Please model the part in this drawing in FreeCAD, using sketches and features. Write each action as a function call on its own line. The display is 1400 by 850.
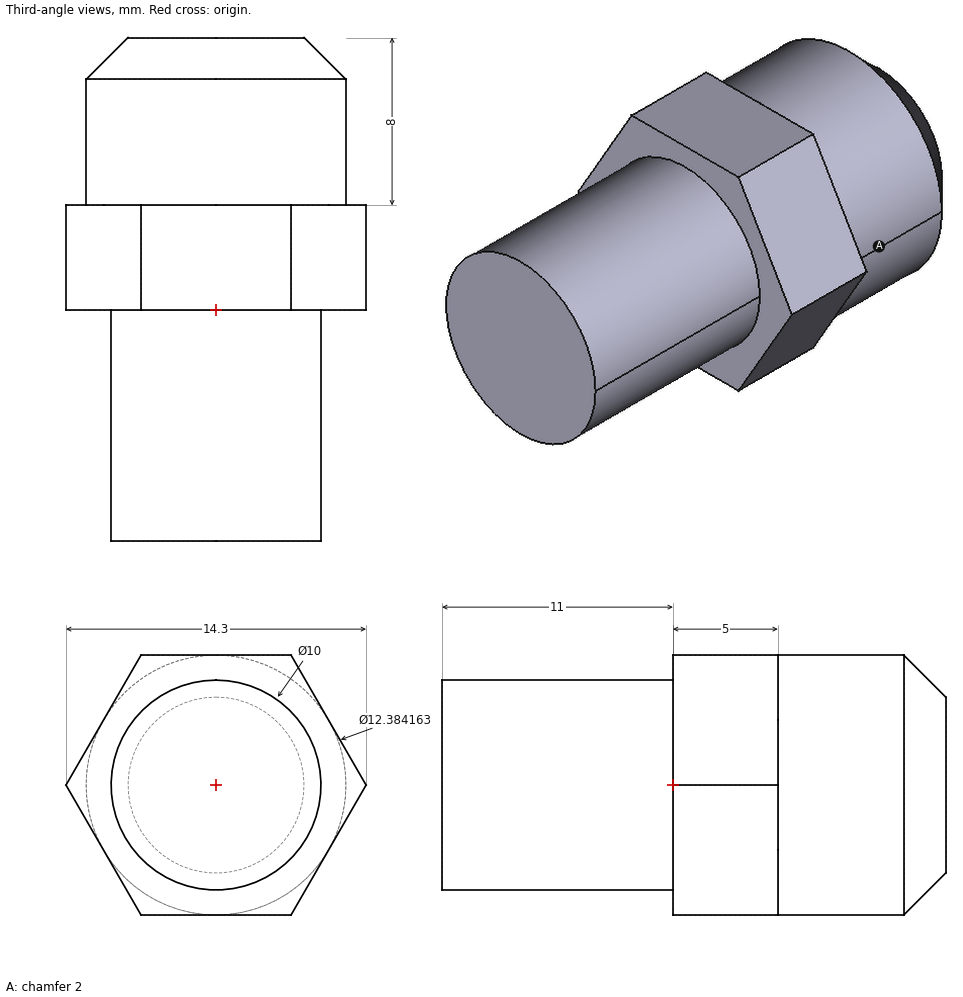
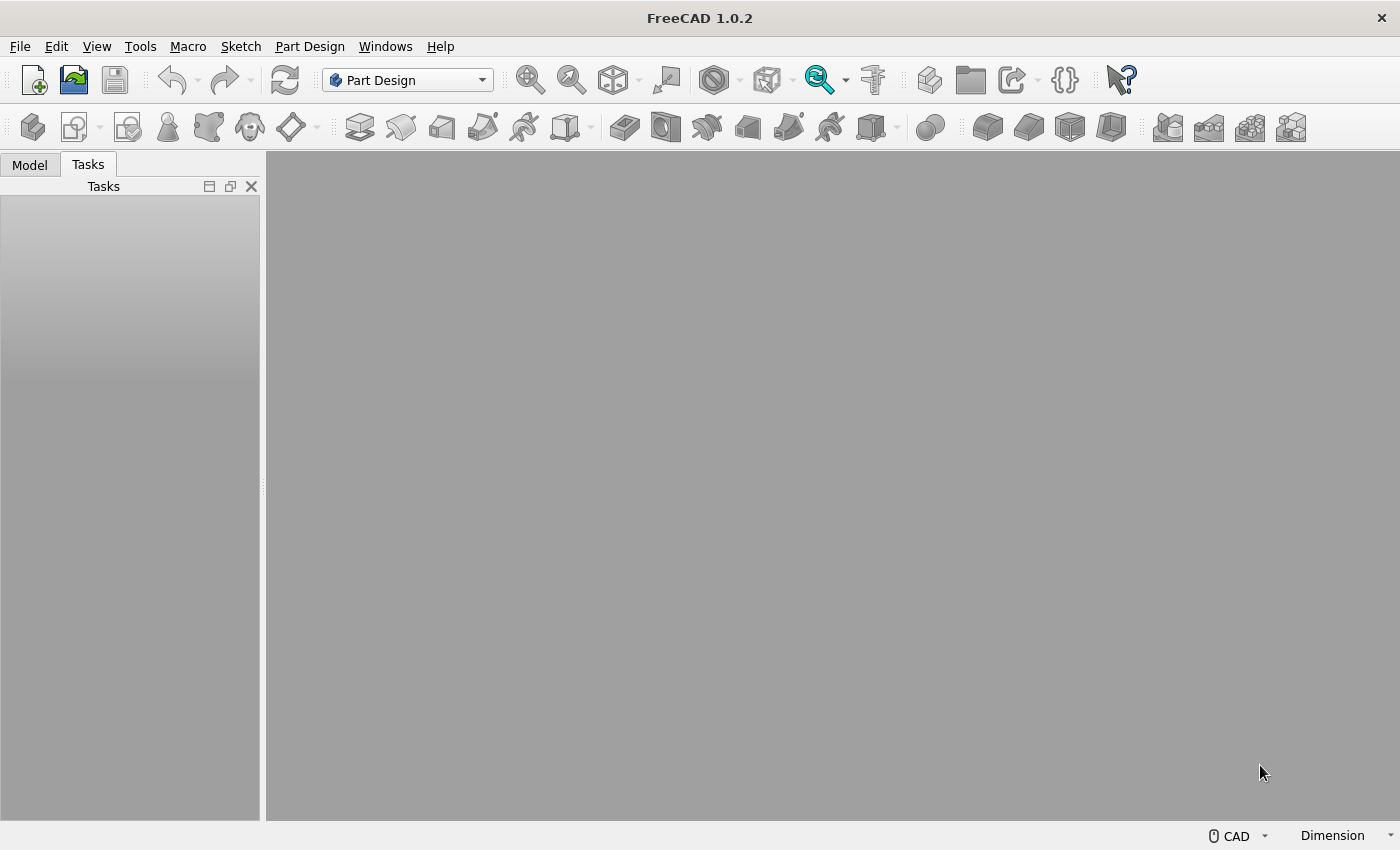
click(33, 80)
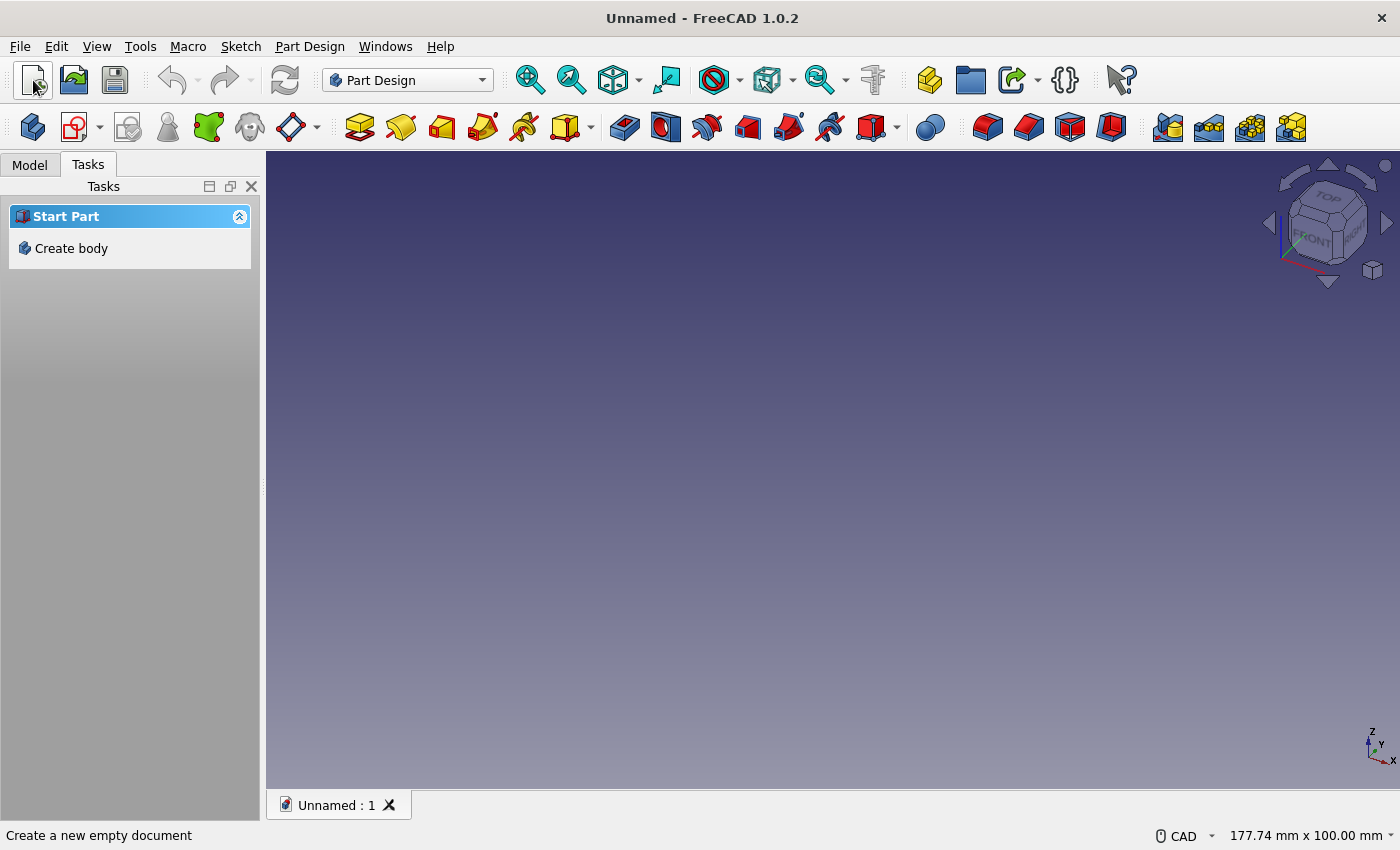
click(74, 128)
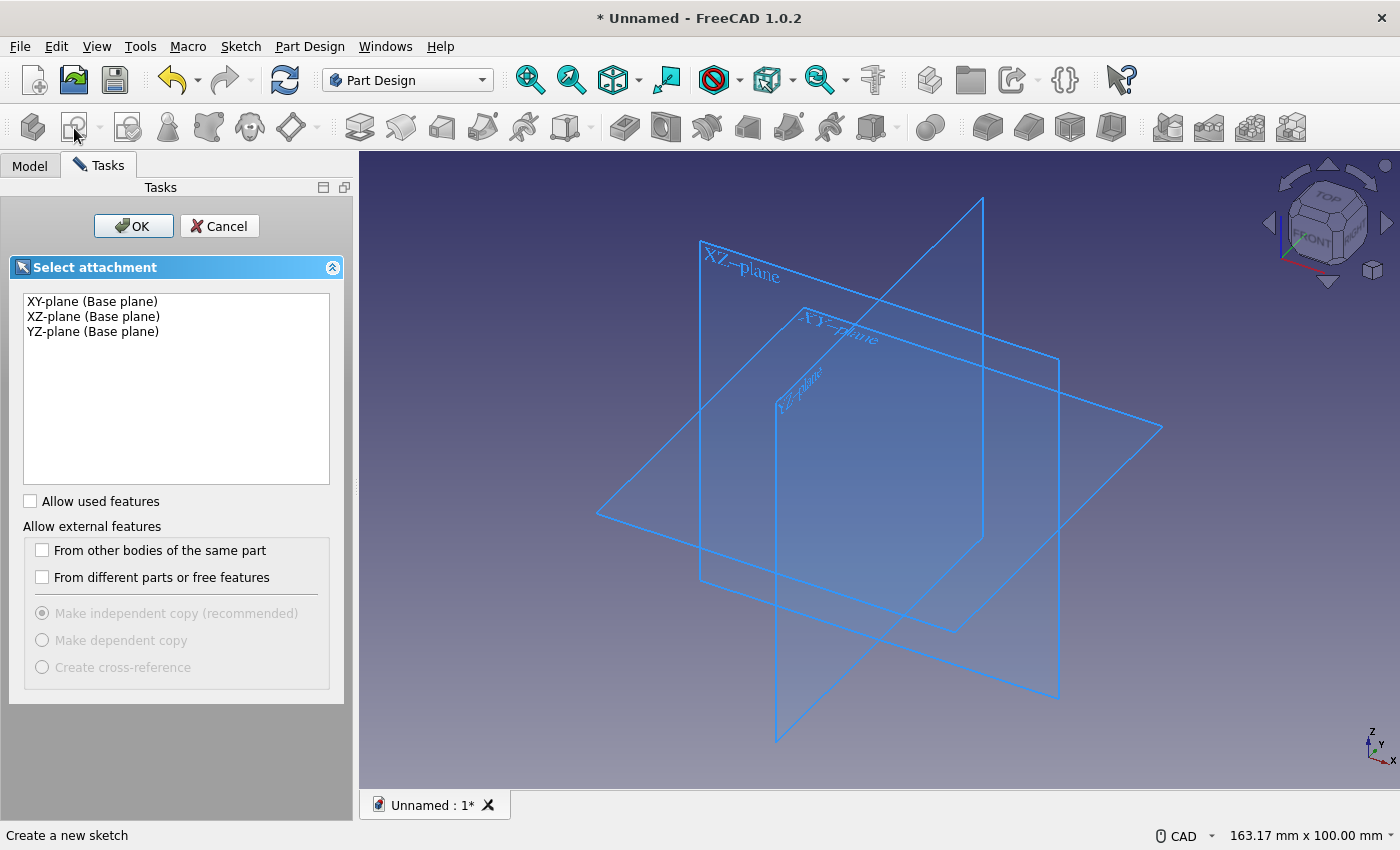
click(84, 316)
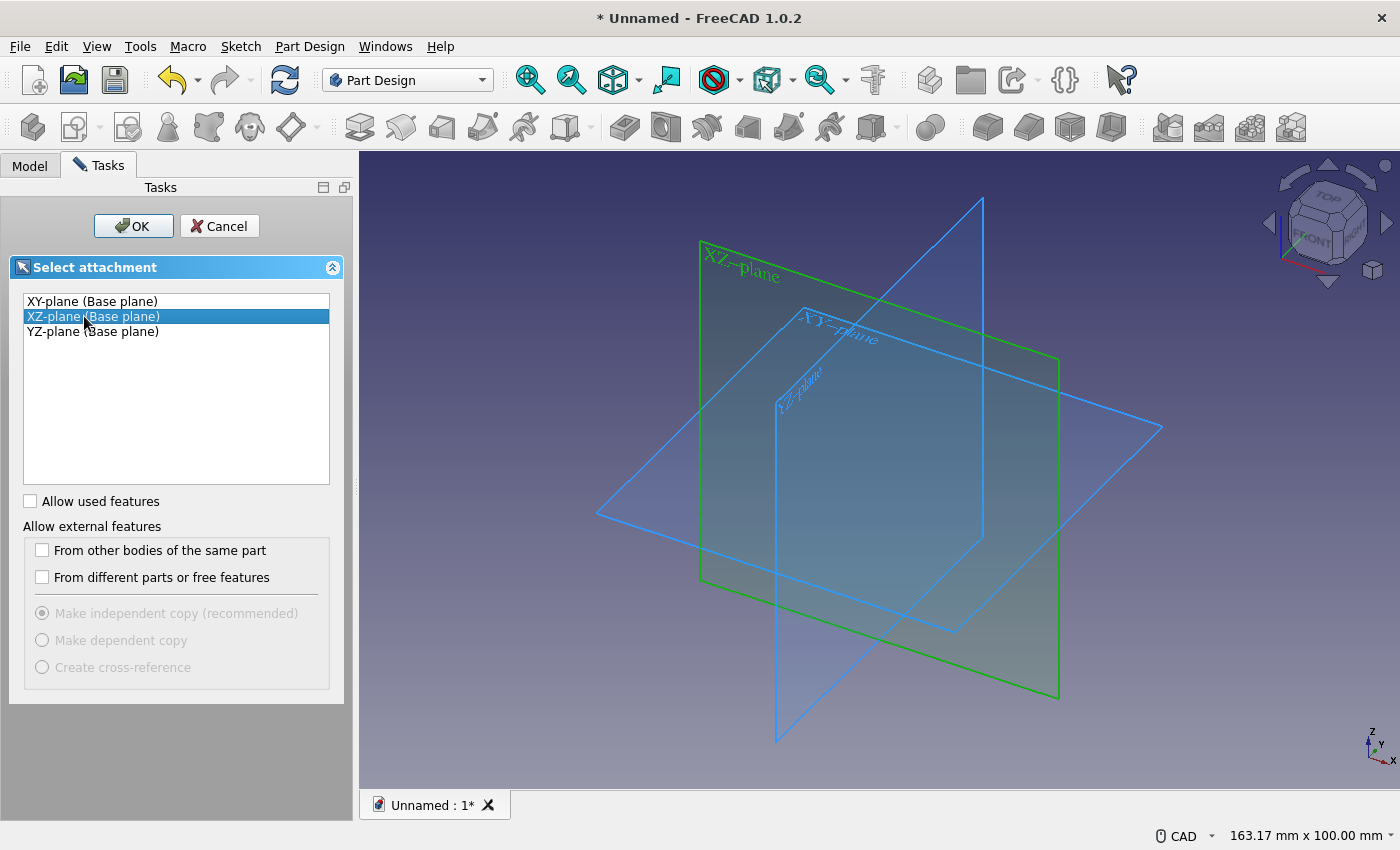
click(134, 226)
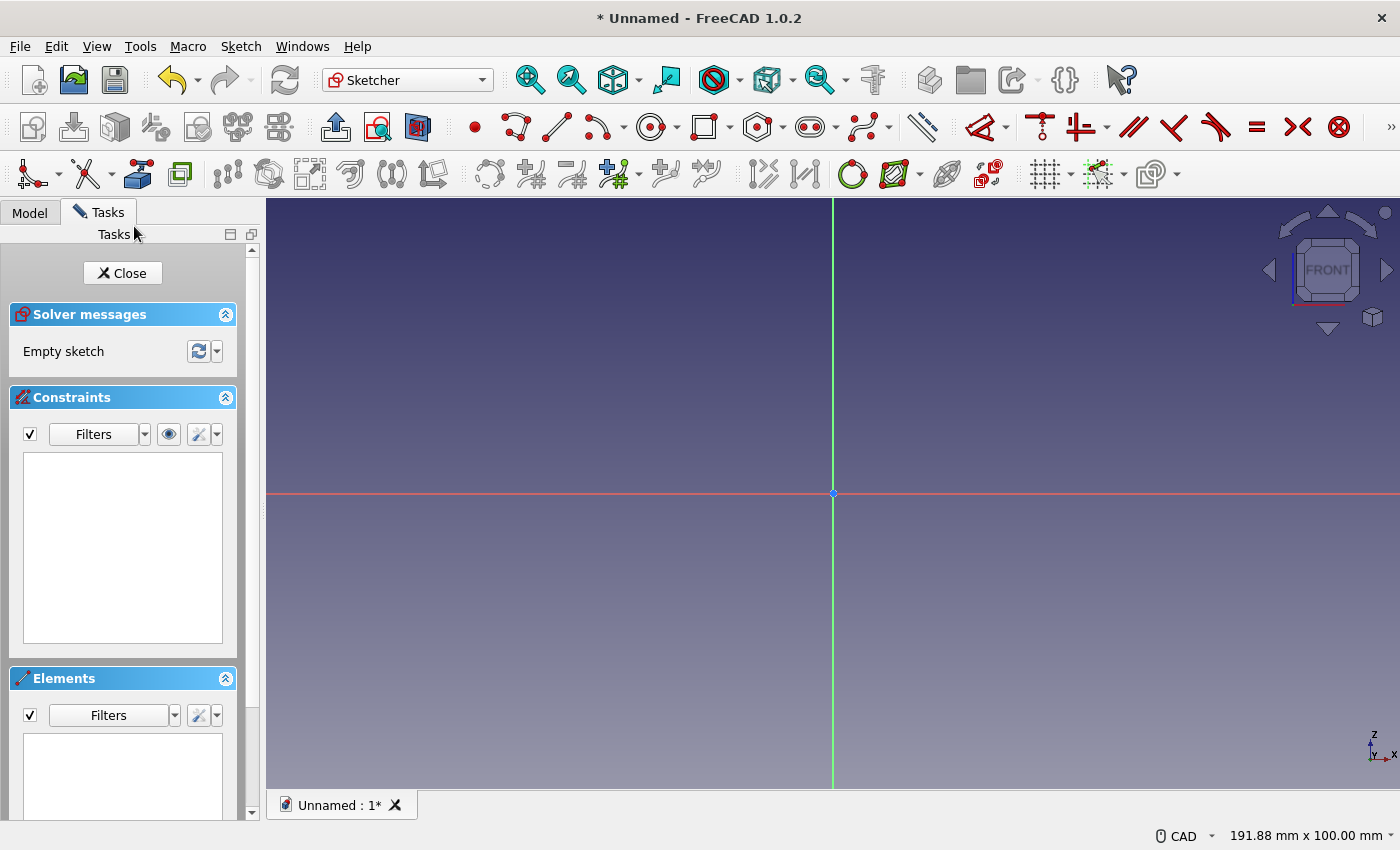
scroll(850, 494, up, 8)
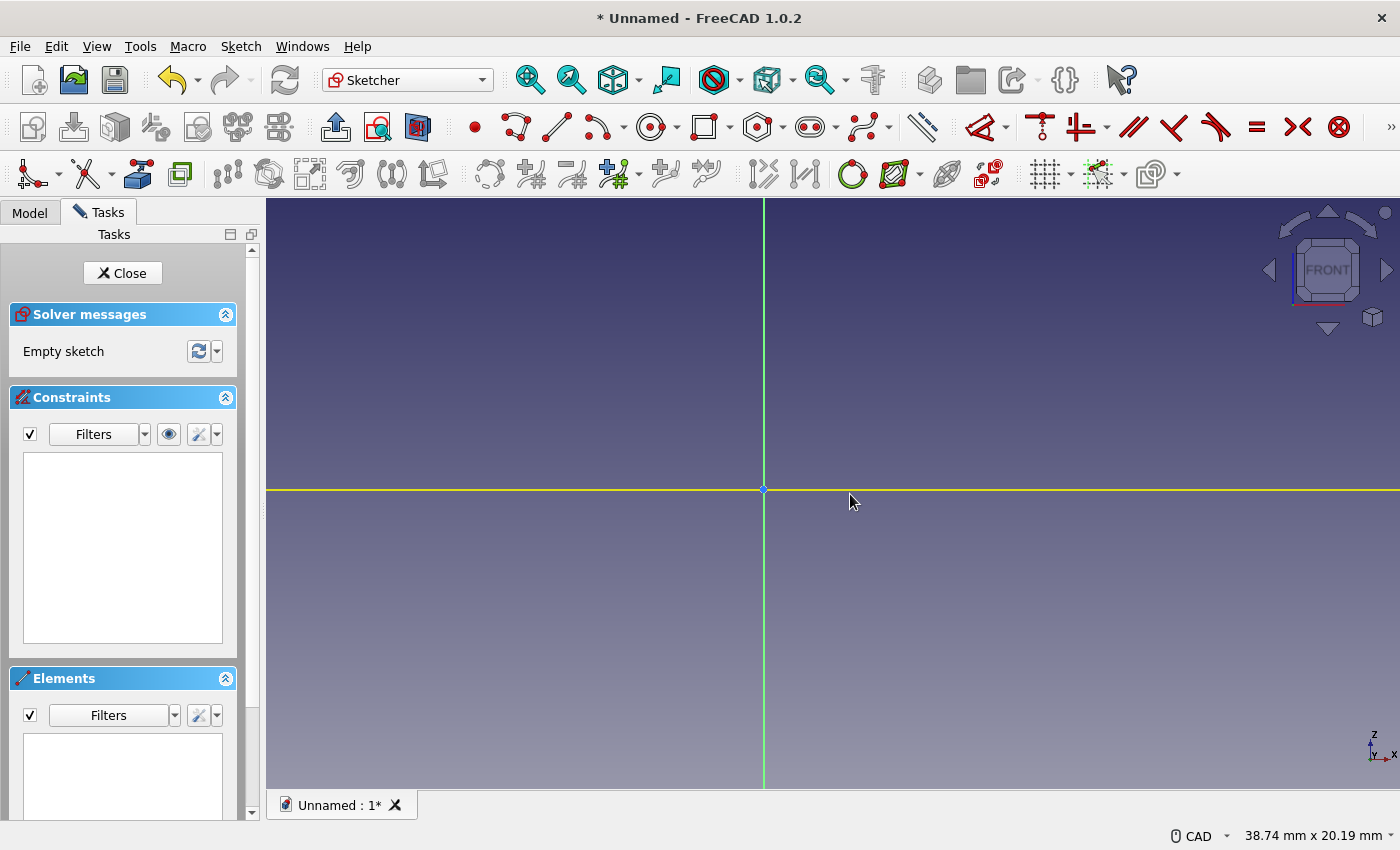
click(756, 128)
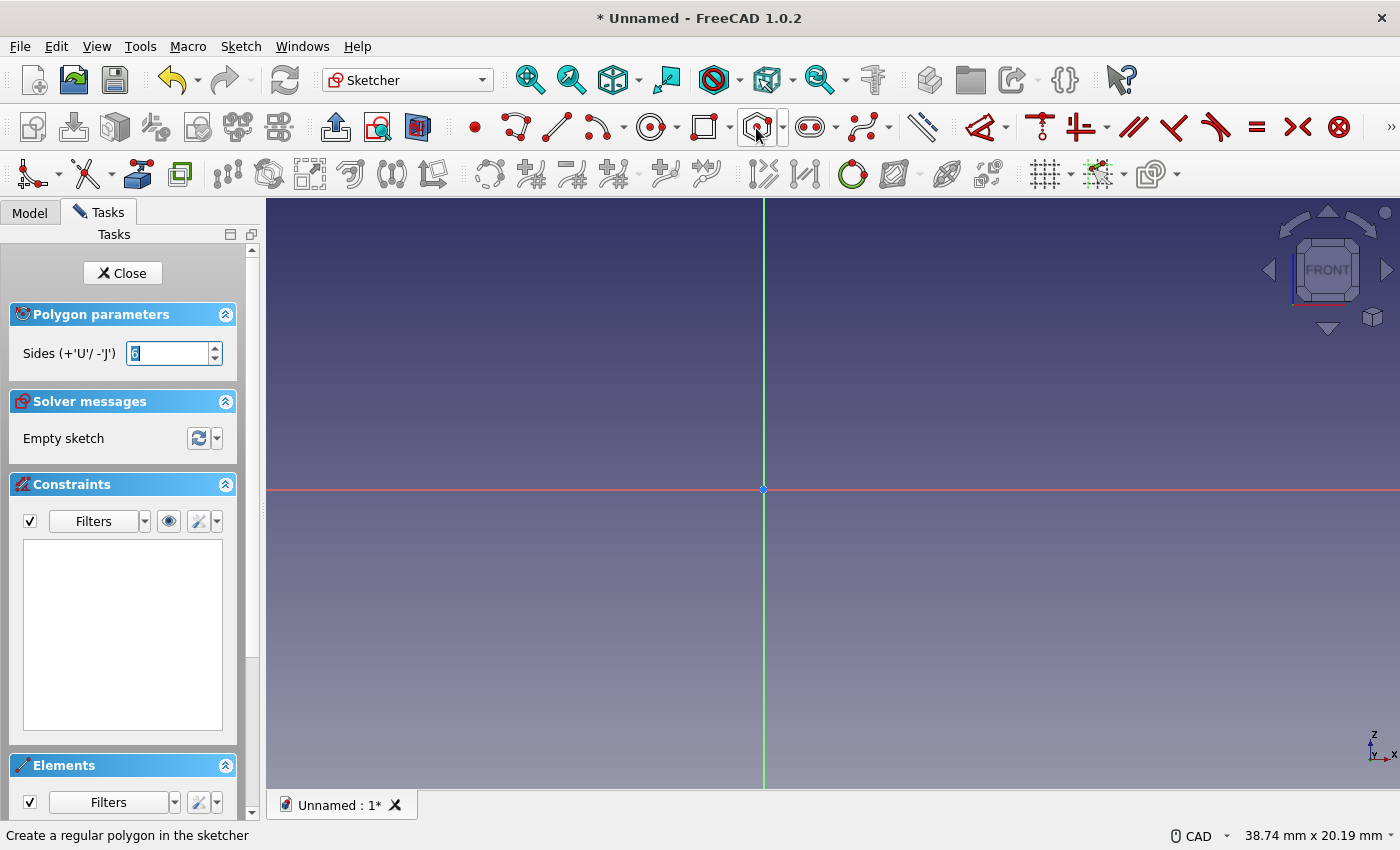
click(764, 490)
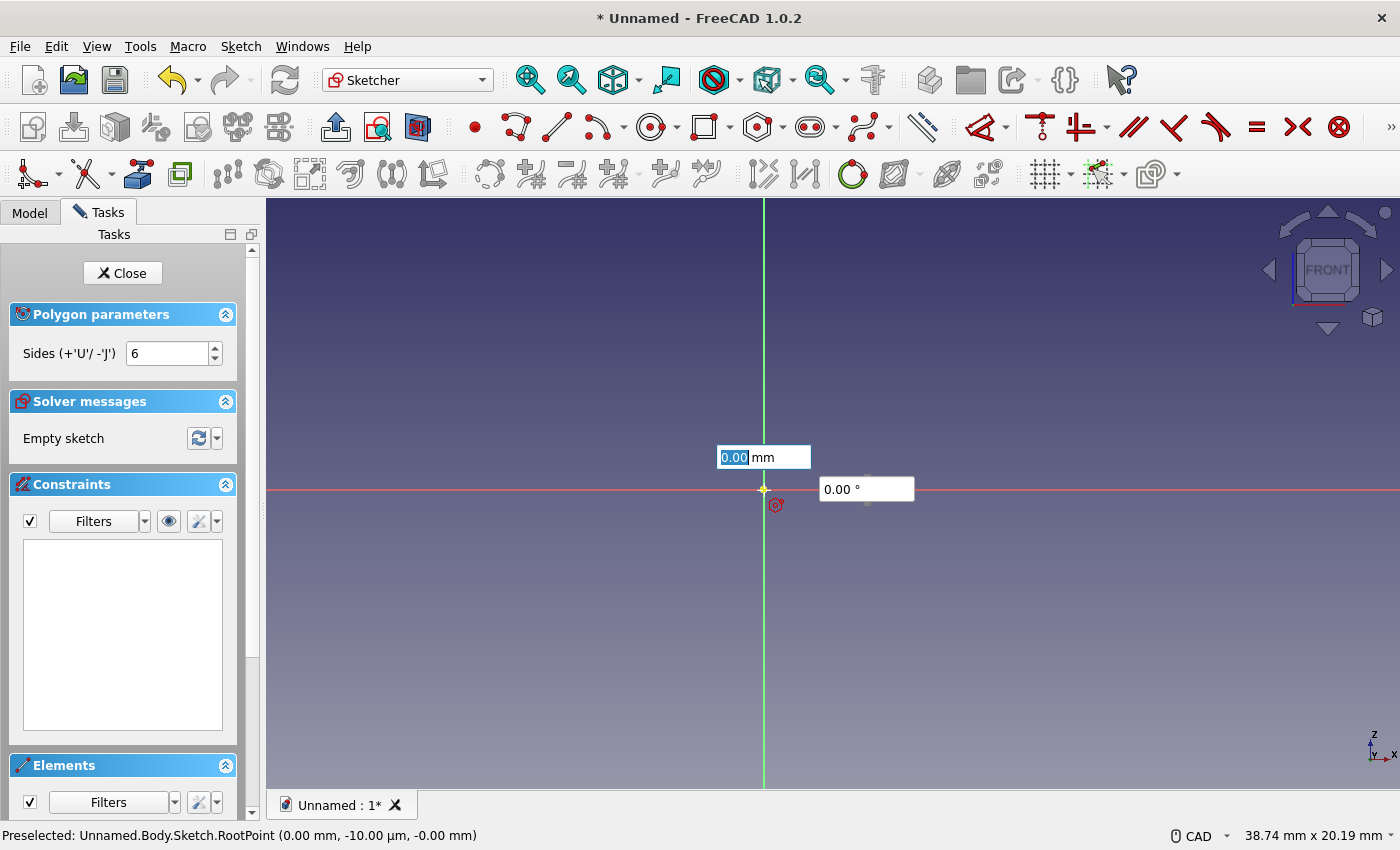
click(554, 490)
right_click(554, 490)